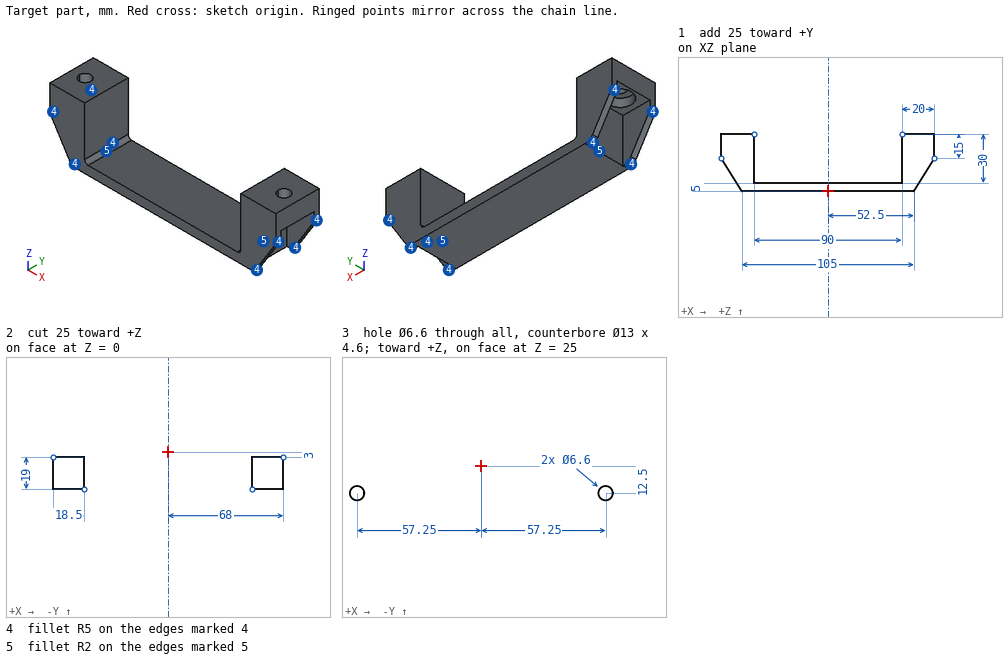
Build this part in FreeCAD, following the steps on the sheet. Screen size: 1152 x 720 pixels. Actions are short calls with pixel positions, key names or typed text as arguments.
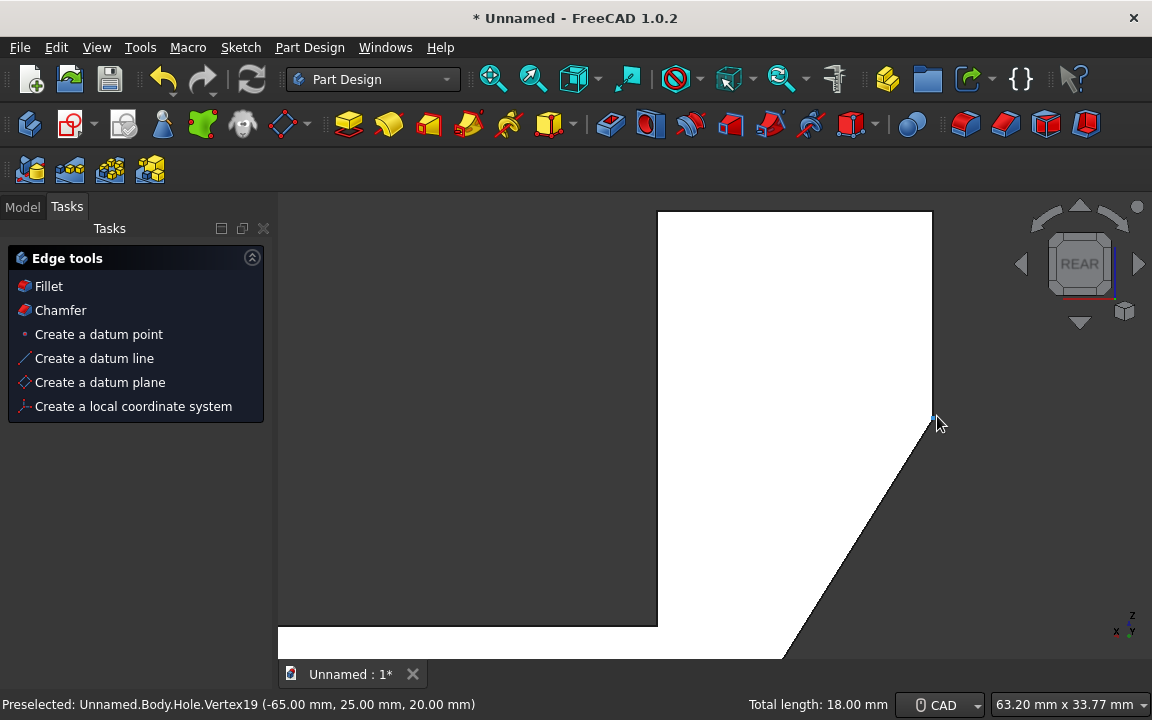
click(494, 80)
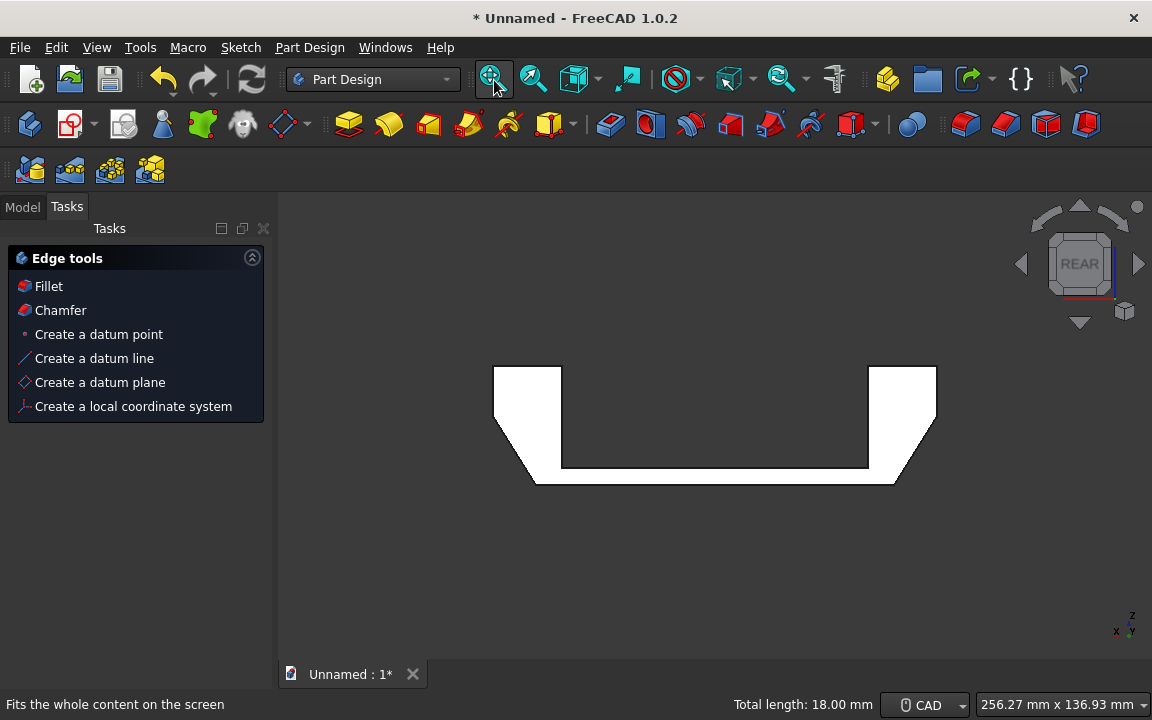
key(6)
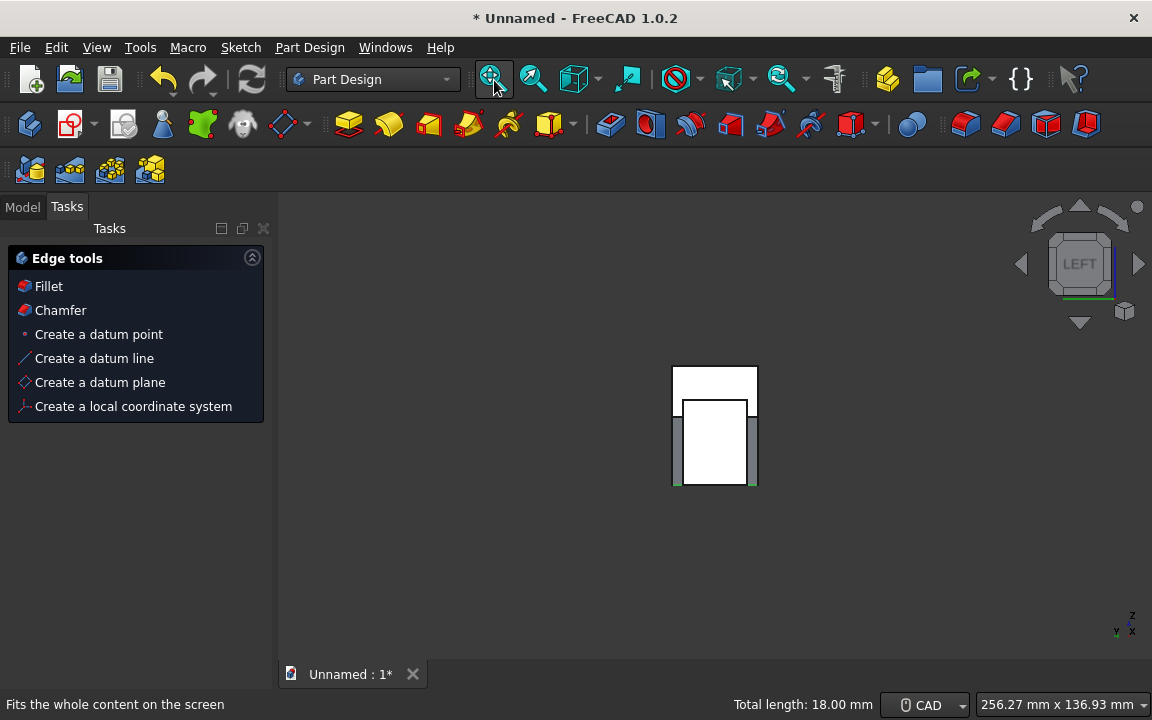
click(494, 80)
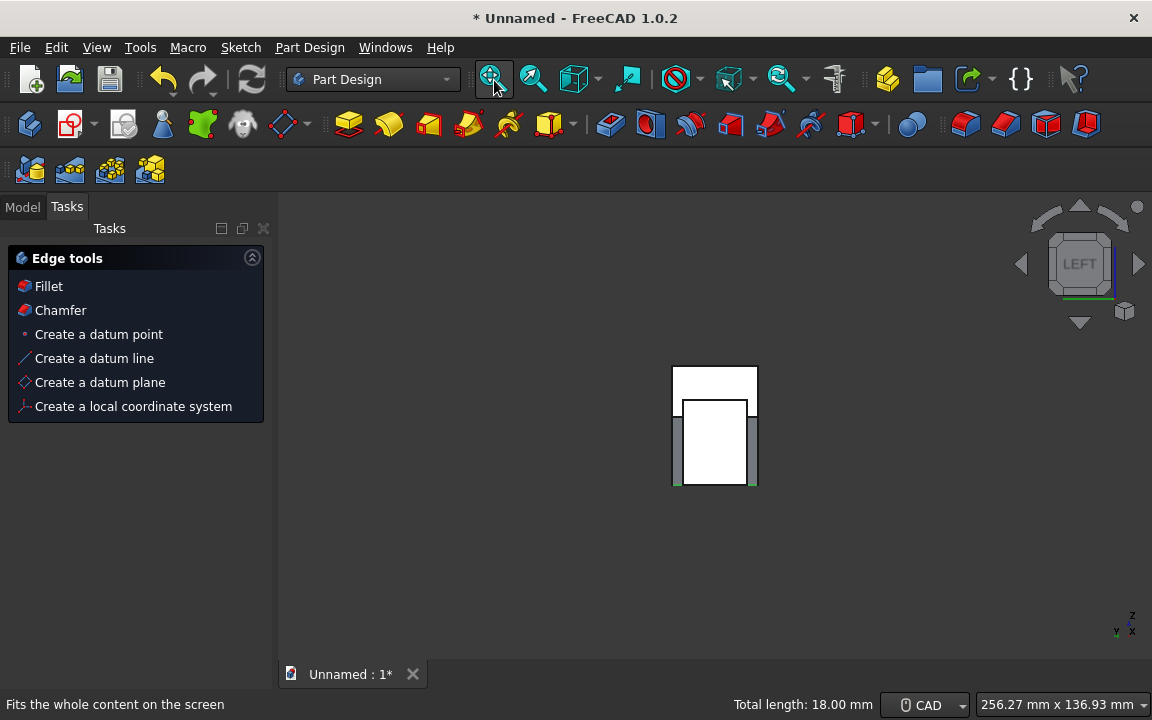
scroll(677, 416, up, 7)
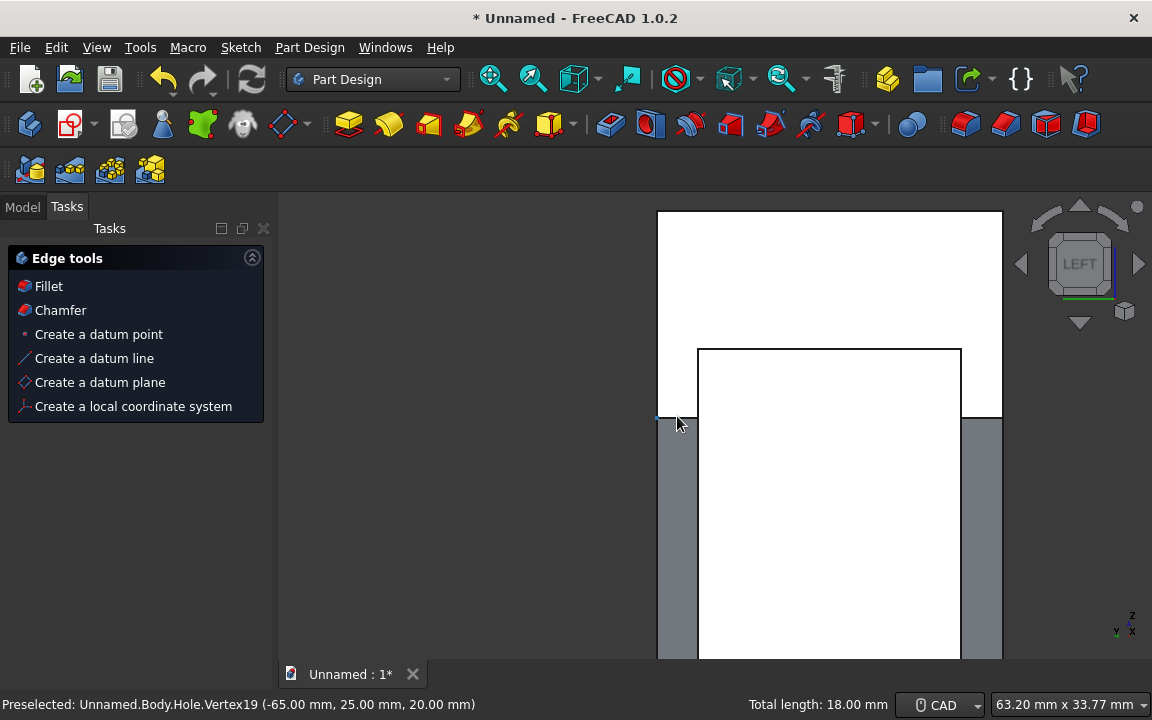
click(678, 417, ctrl)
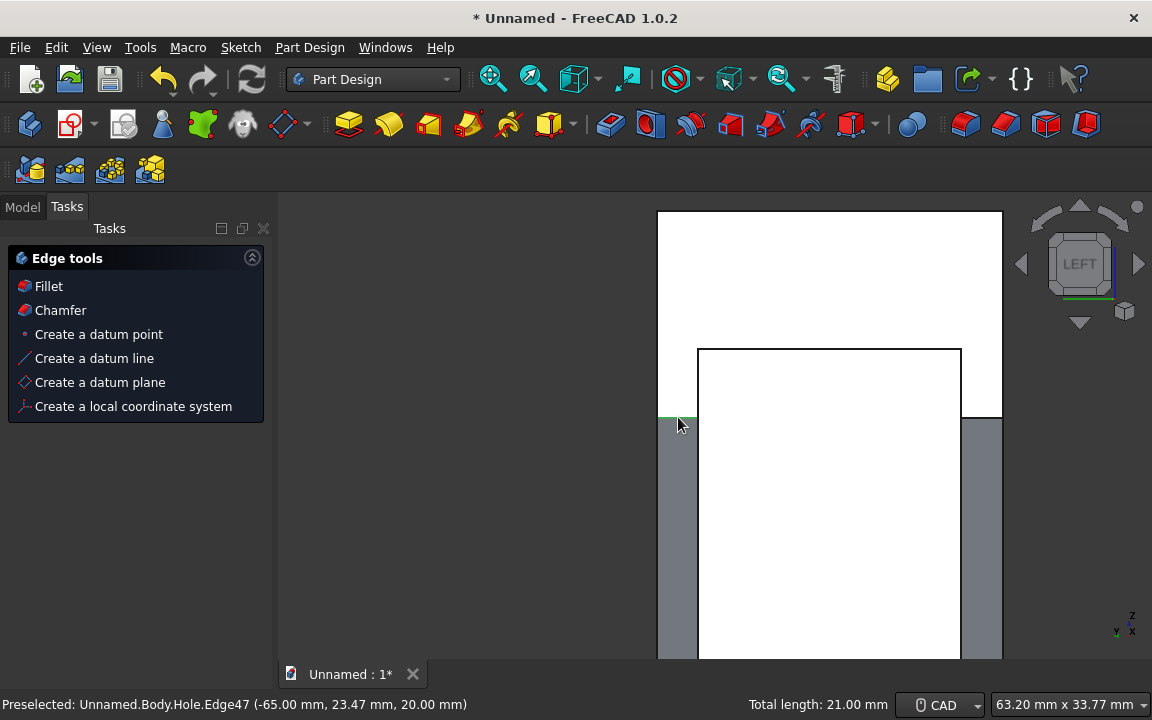
click(982, 417, ctrl)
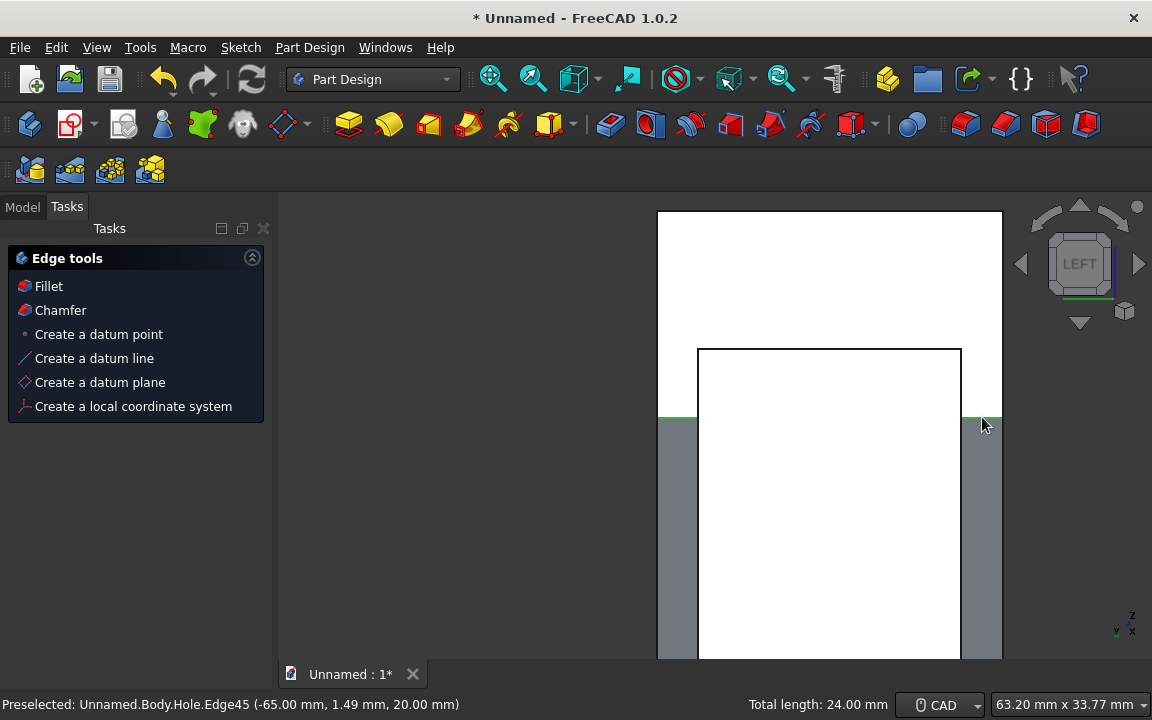
click(966, 124)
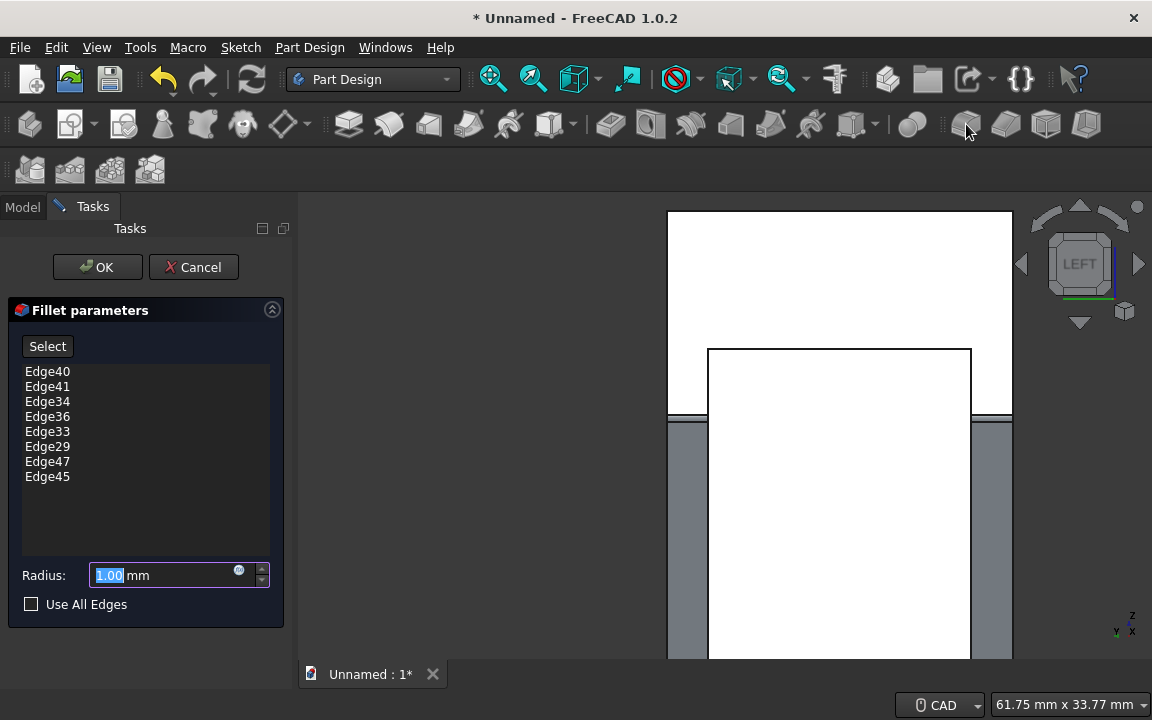
text(5)
key(Tab)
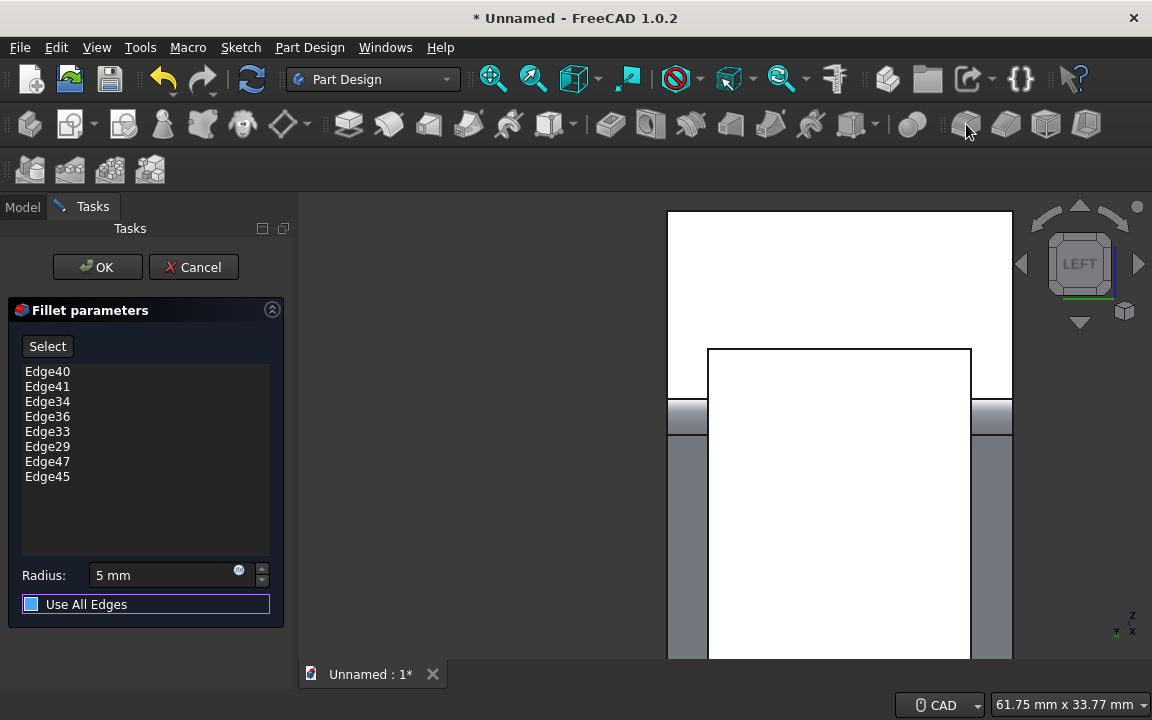
click(98, 267)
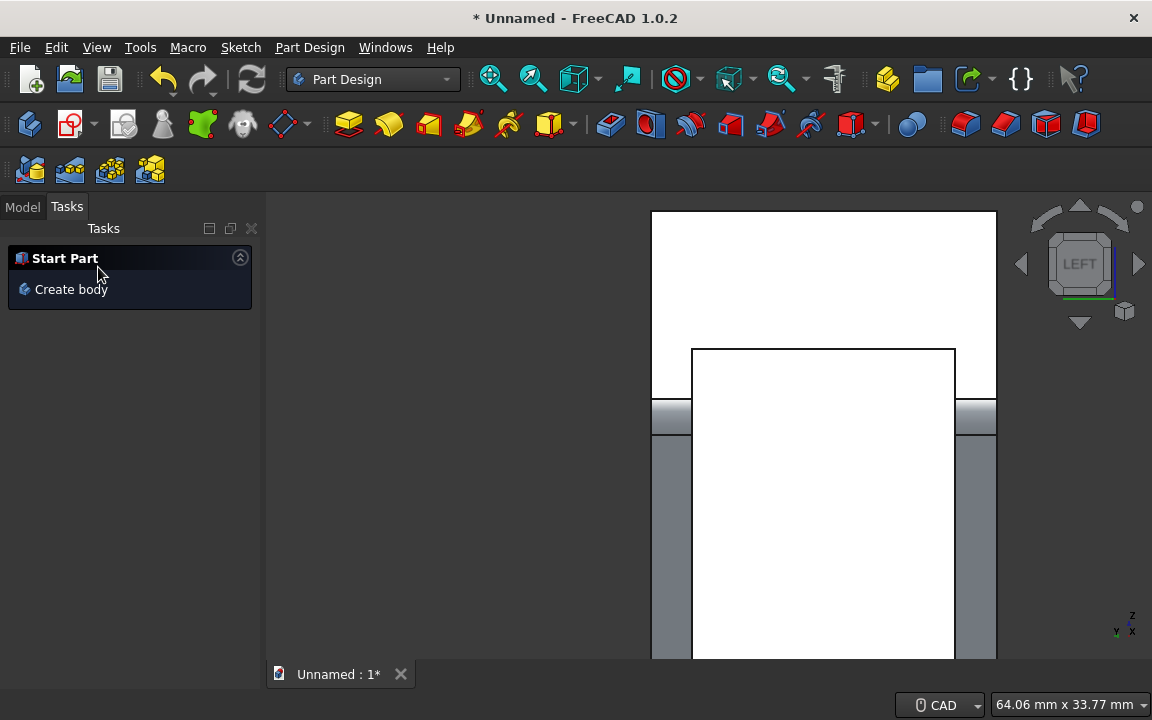
click(494, 80)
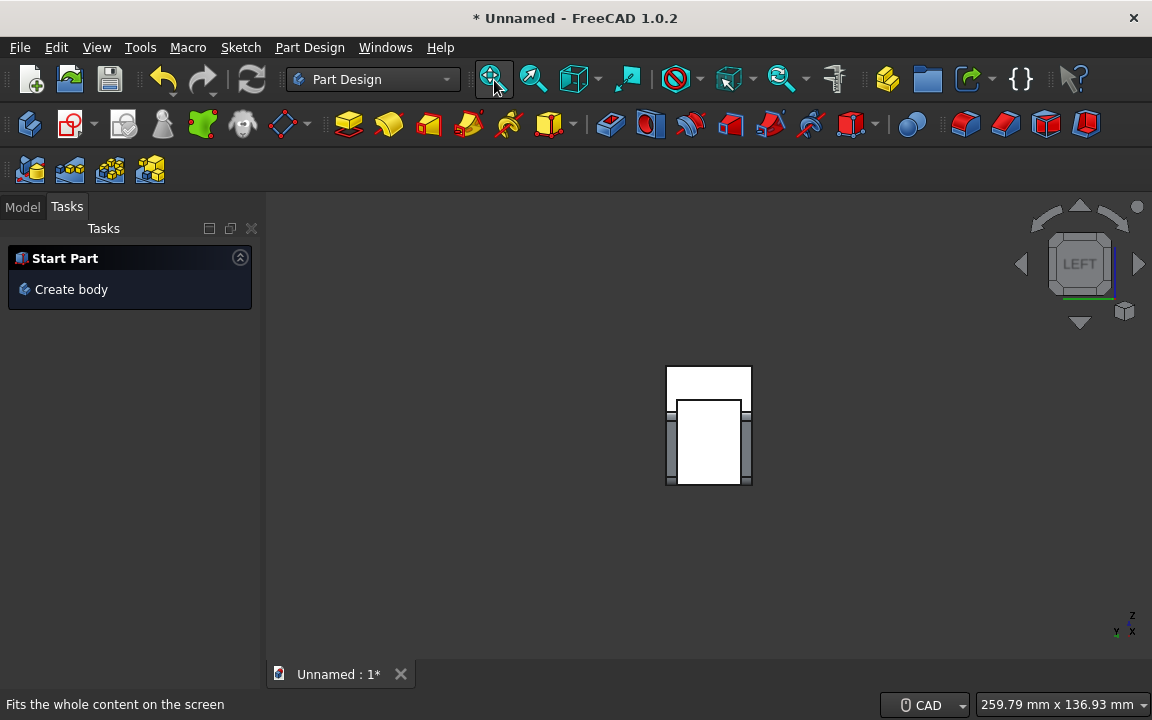
key(0)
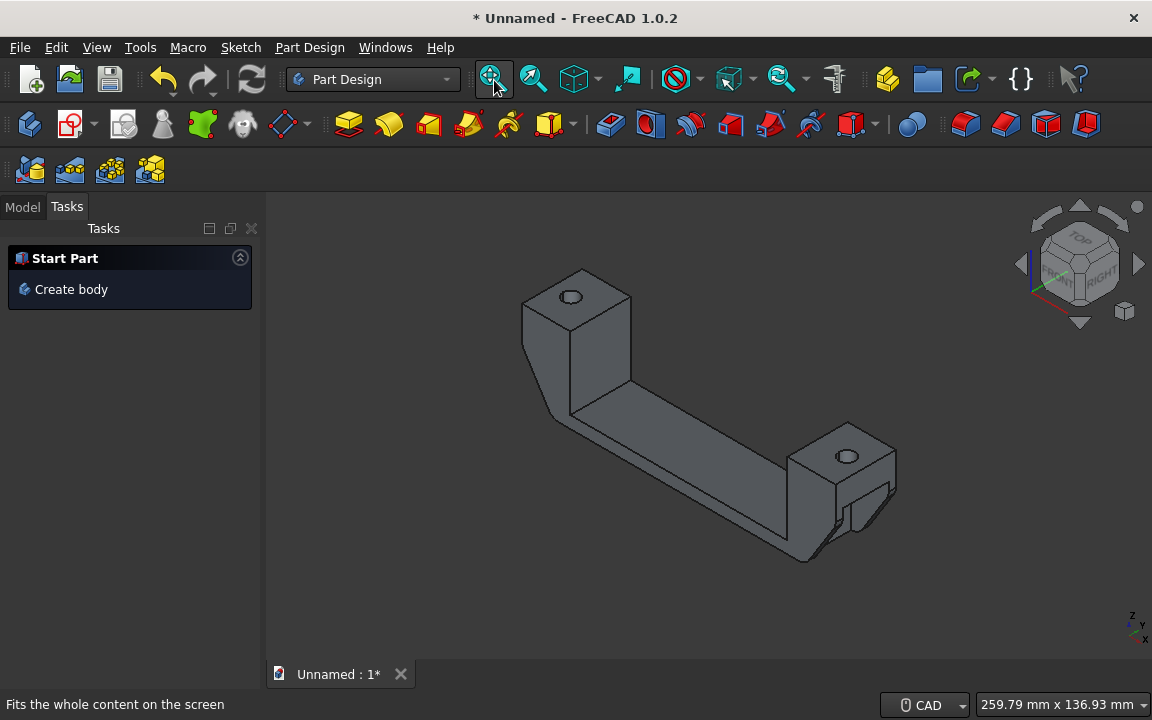
key(2)